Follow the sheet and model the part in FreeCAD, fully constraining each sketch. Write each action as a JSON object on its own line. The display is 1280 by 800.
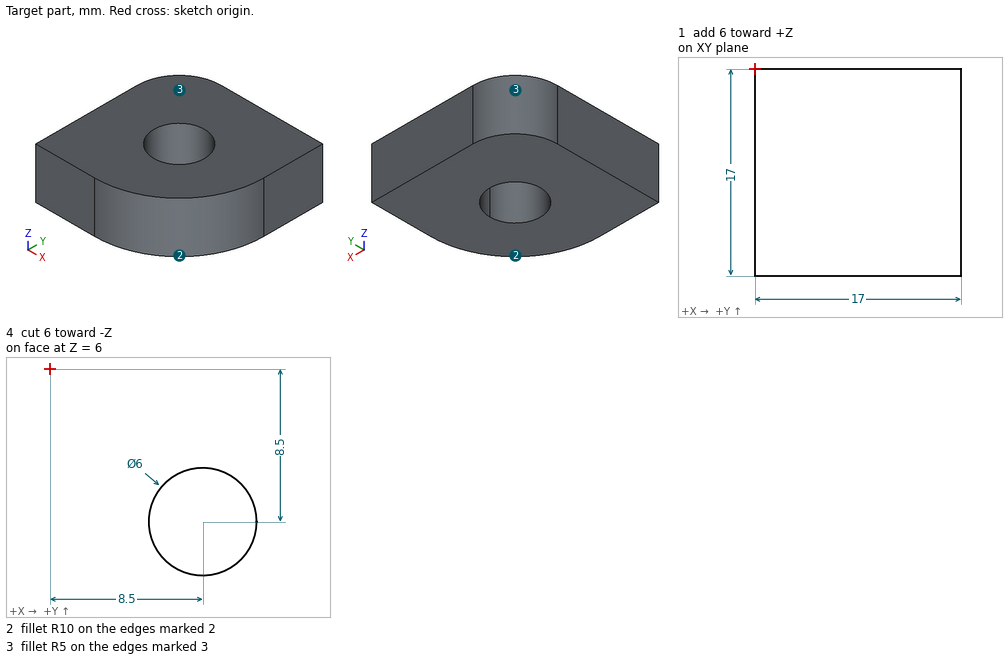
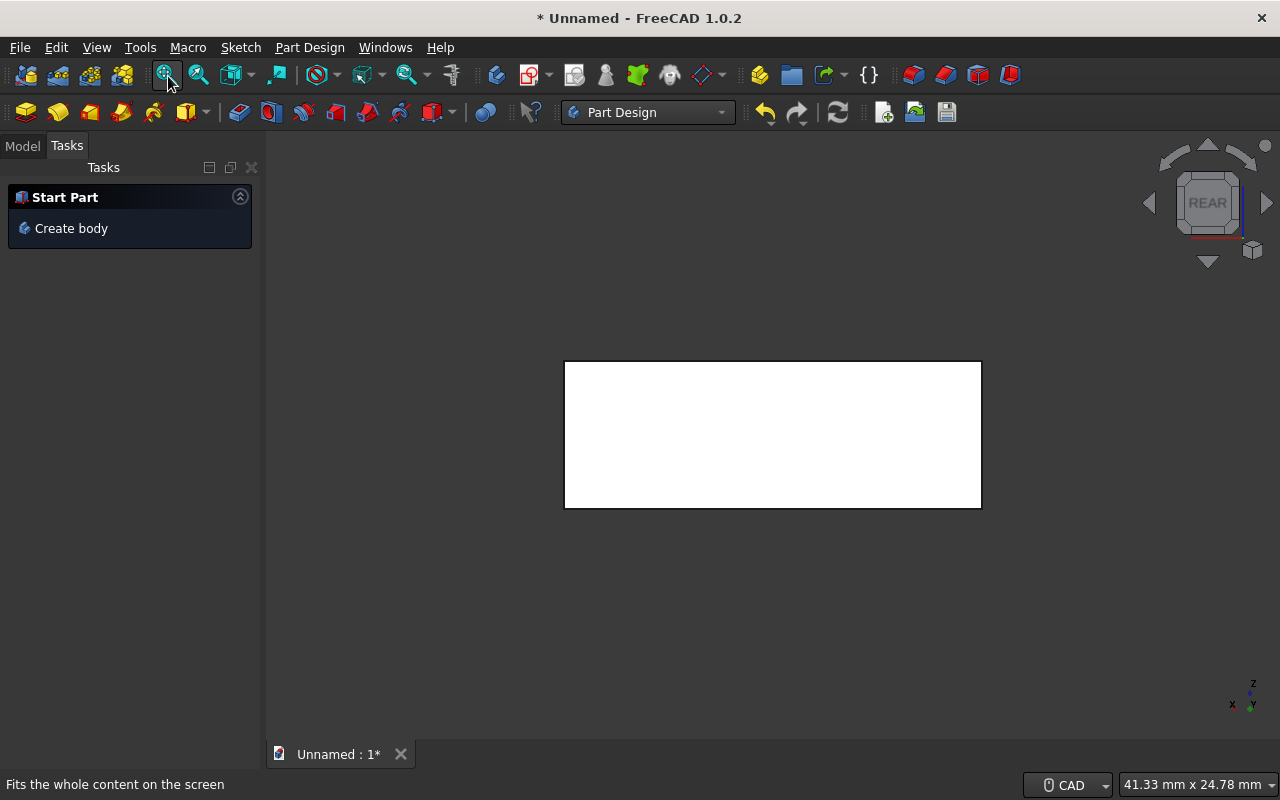
{"action": "left_click", "coordinate": [168, 76]}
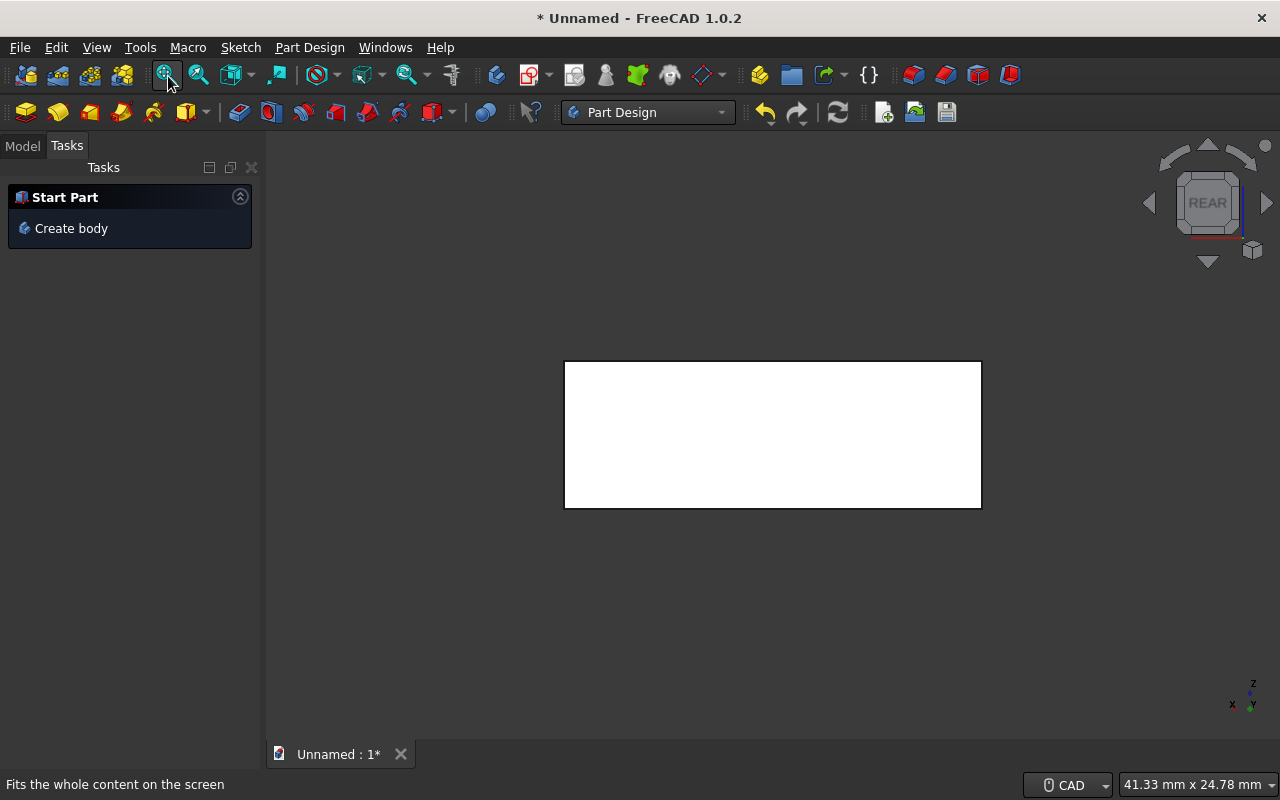
{"action": "left_click", "coordinate": [982, 434]}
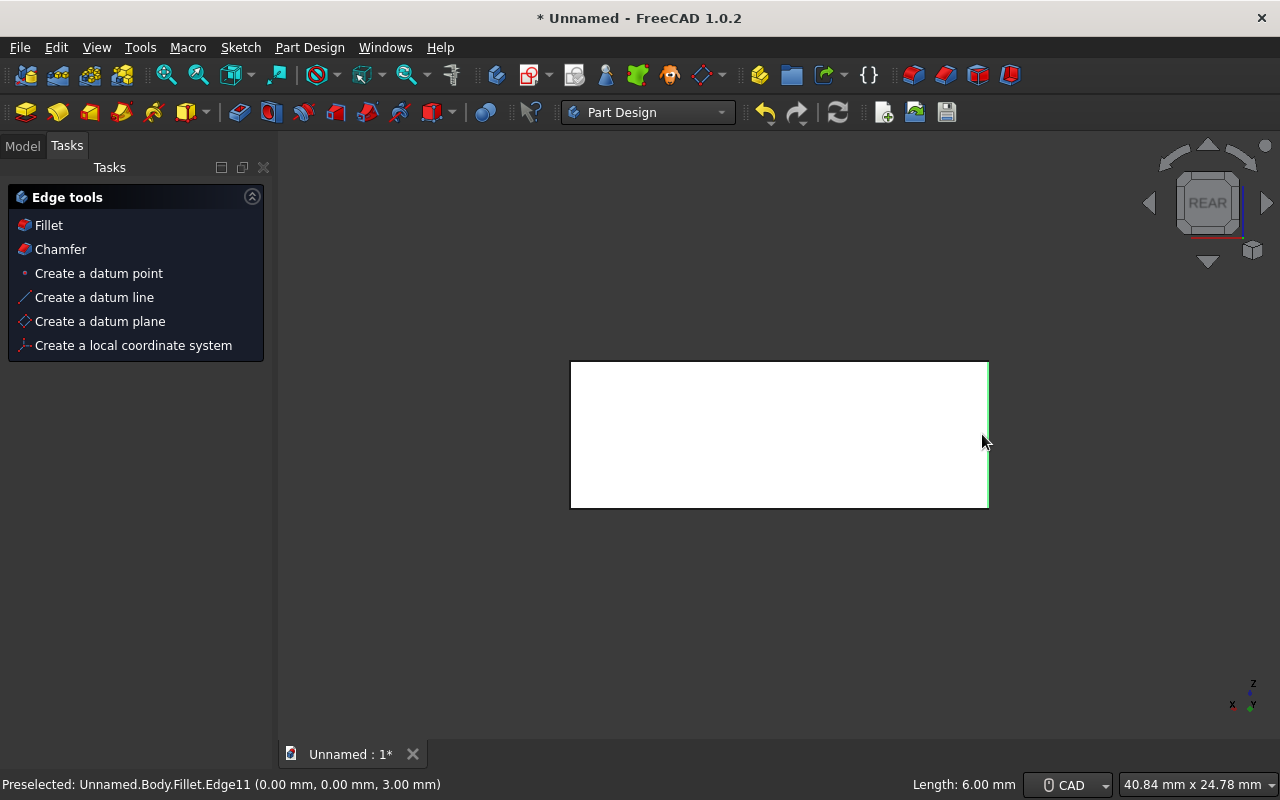
{"action": "left_click", "coordinate": [914, 76]}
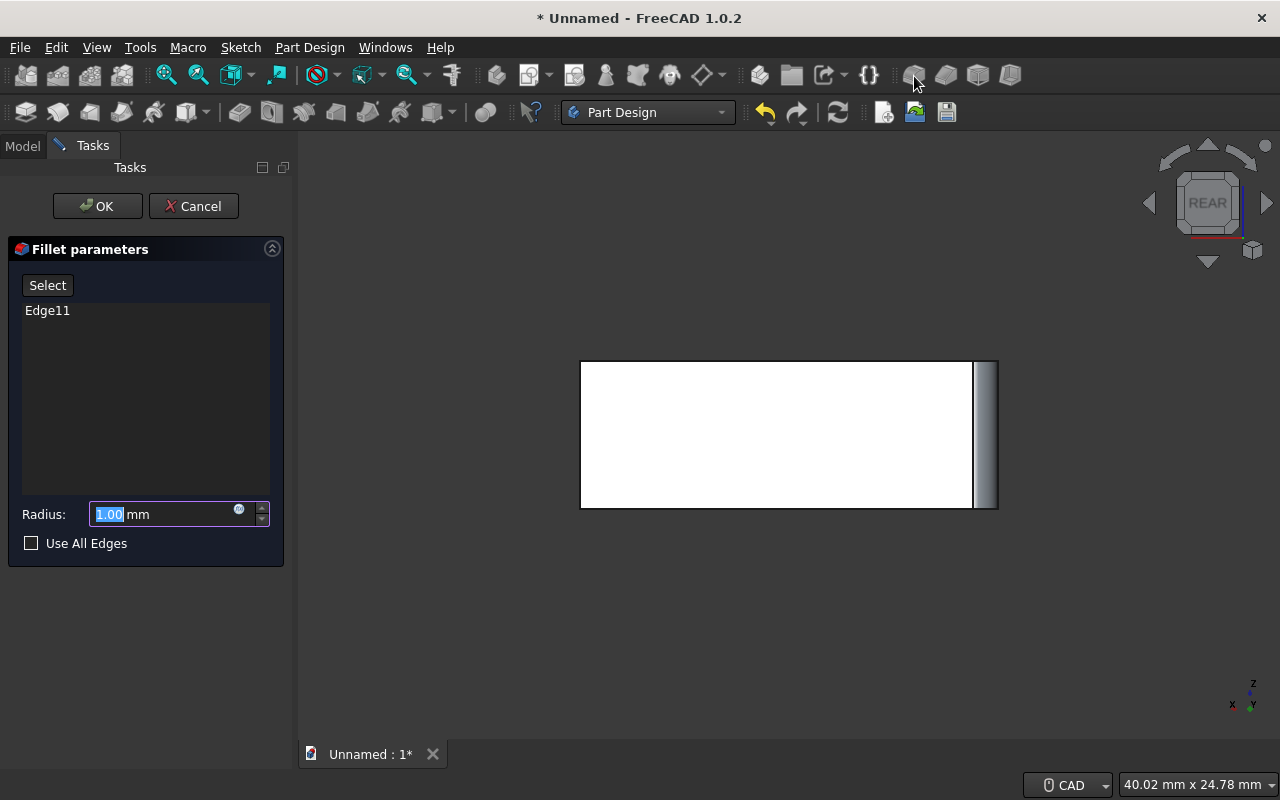
{"action": "type", "text": "5"}
{"action": "key", "text": "Tab"}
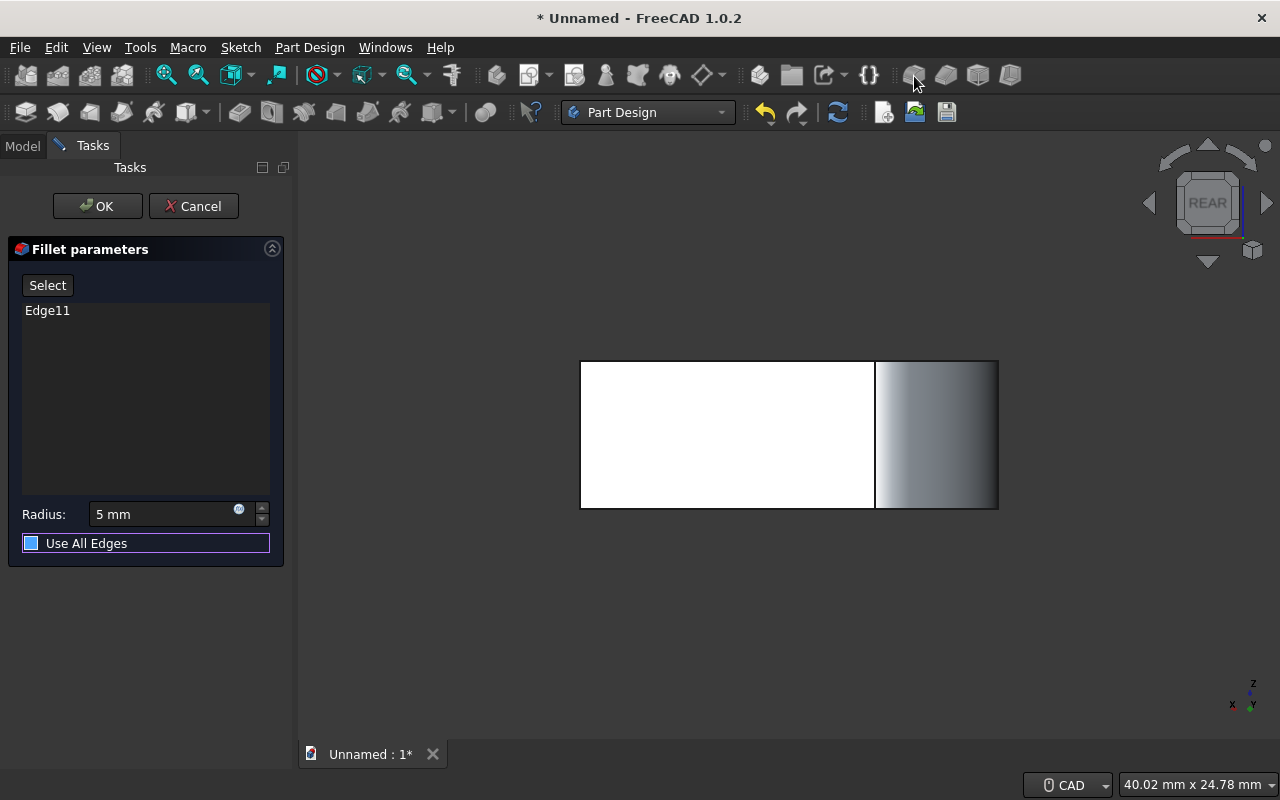
{"action": "left_click", "coordinate": [98, 206]}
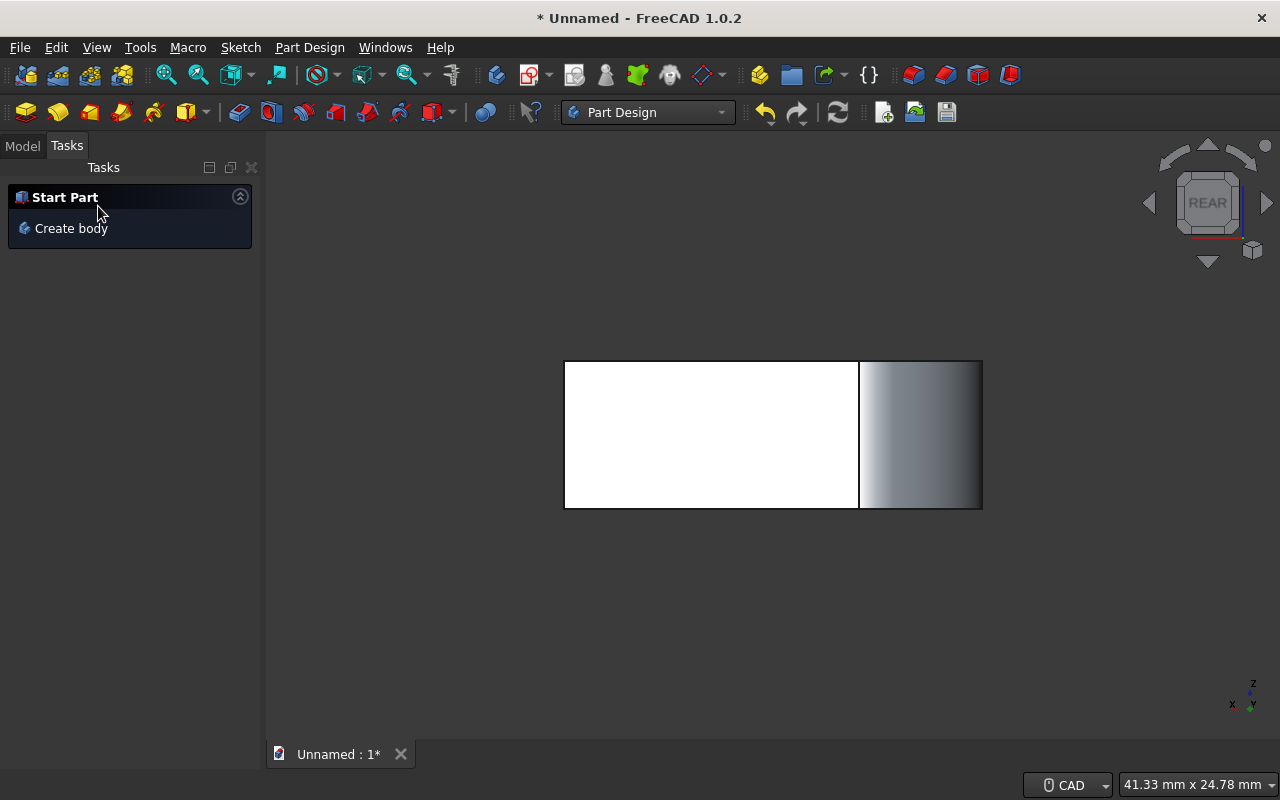
{"action": "key", "text": "v f"}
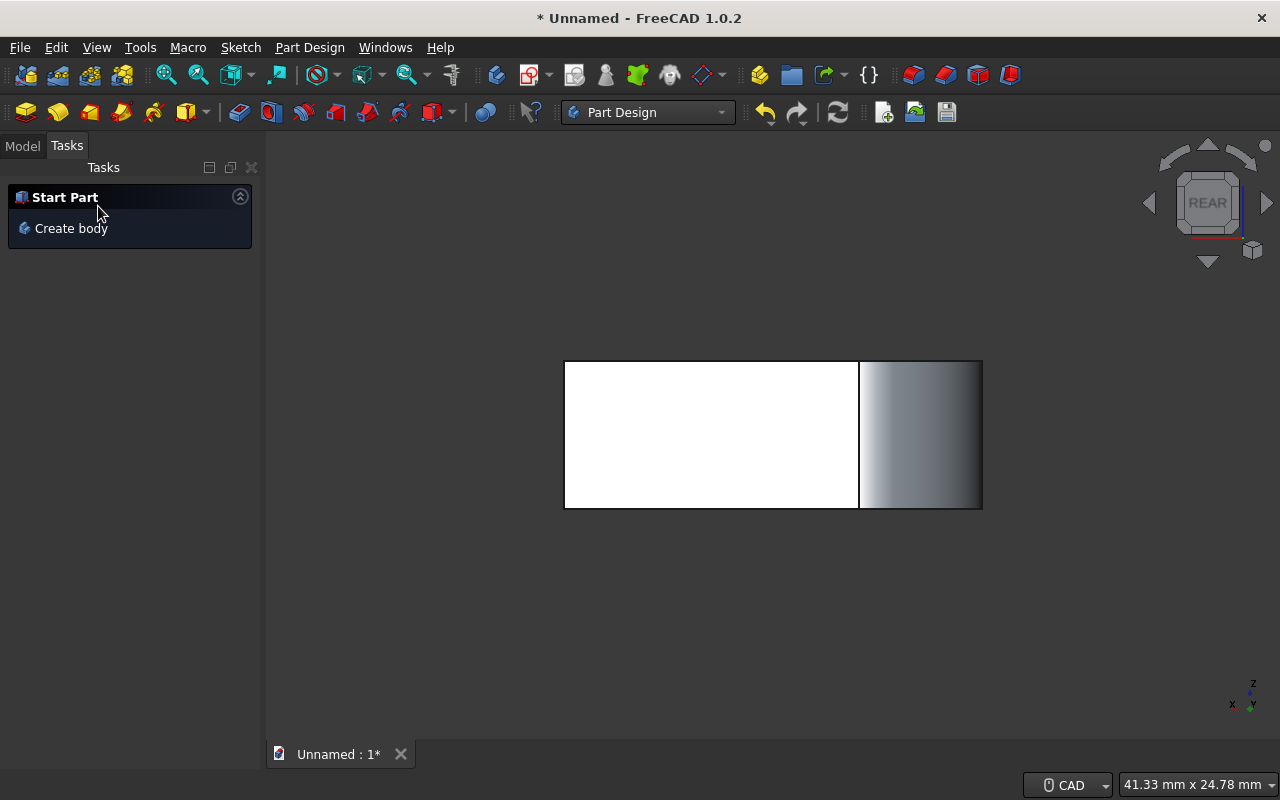
{"action": "key", "text": "0"}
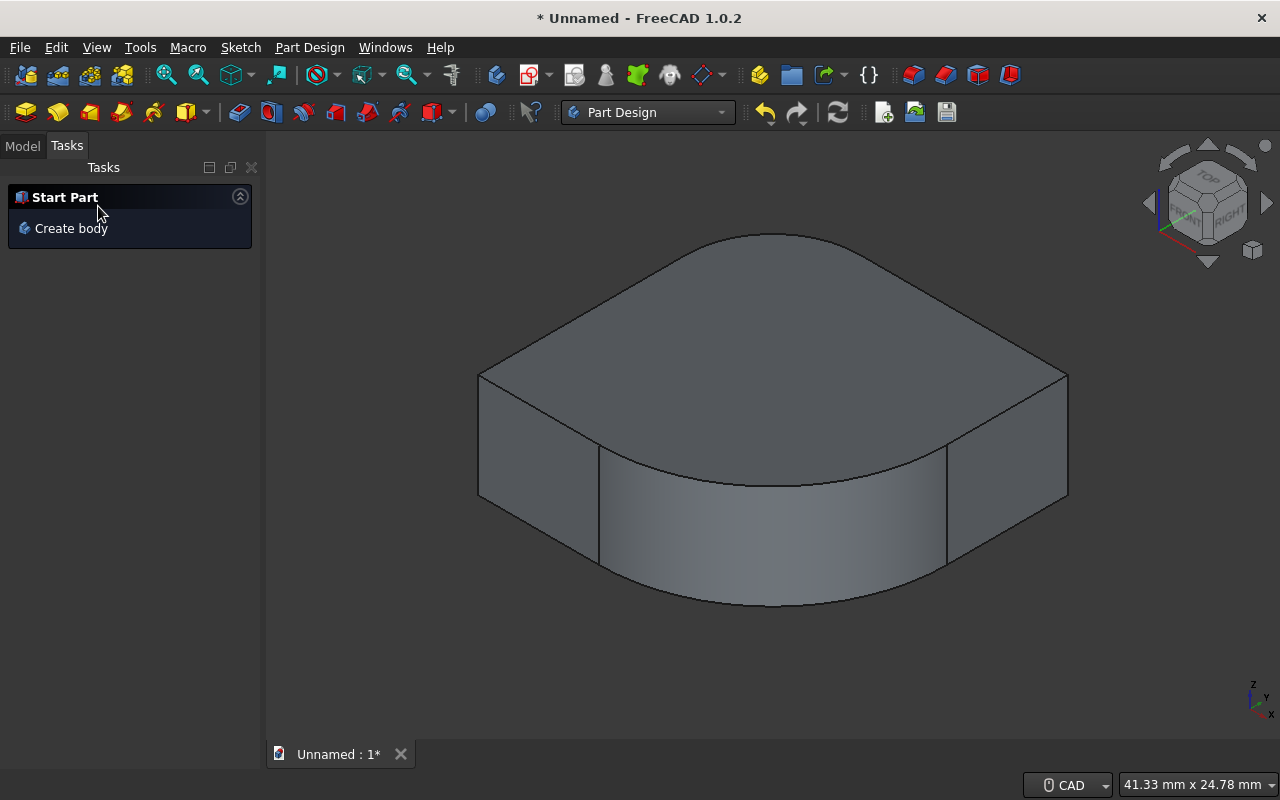
{"action": "left_click", "coordinate": [773, 374]}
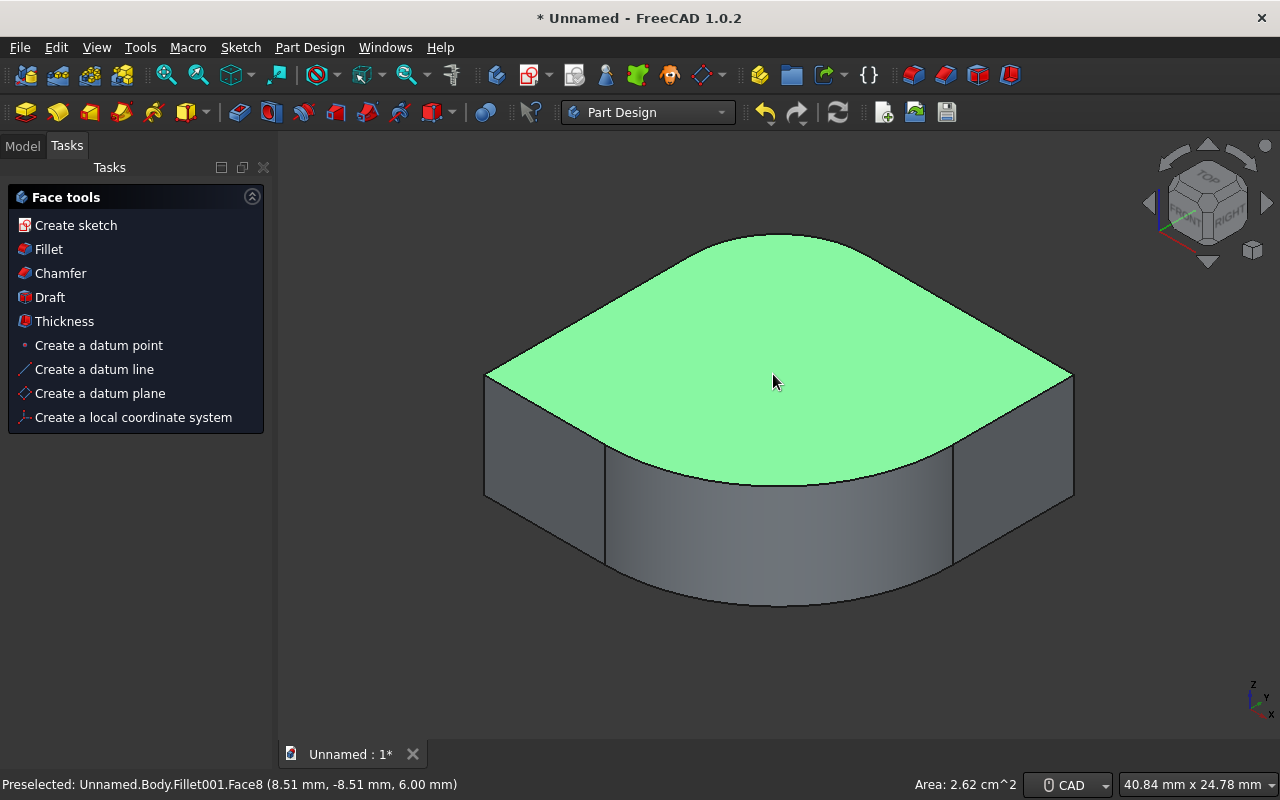
{"action": "left_click", "coordinate": [530, 76]}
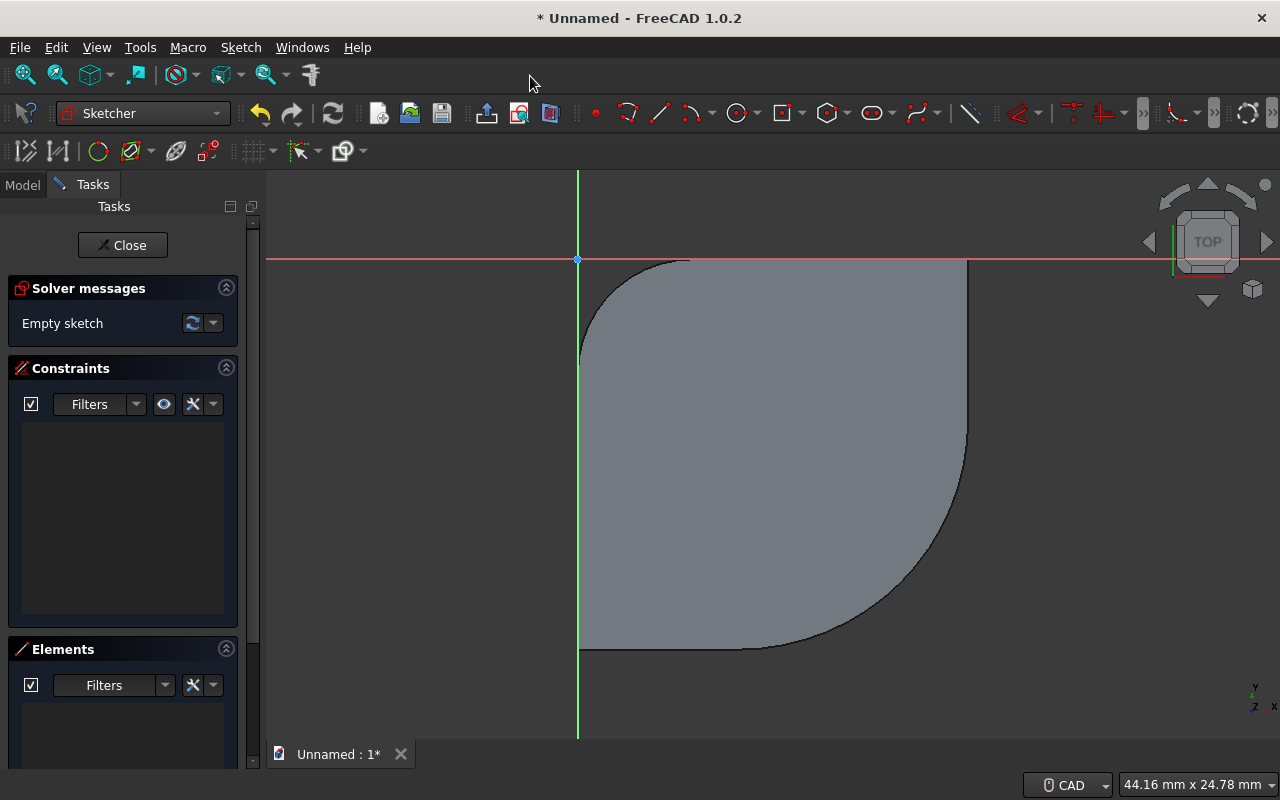
{"action": "scroll", "coordinate": [721, 263], "scroll_direction": "up", "scroll_amount": 2}